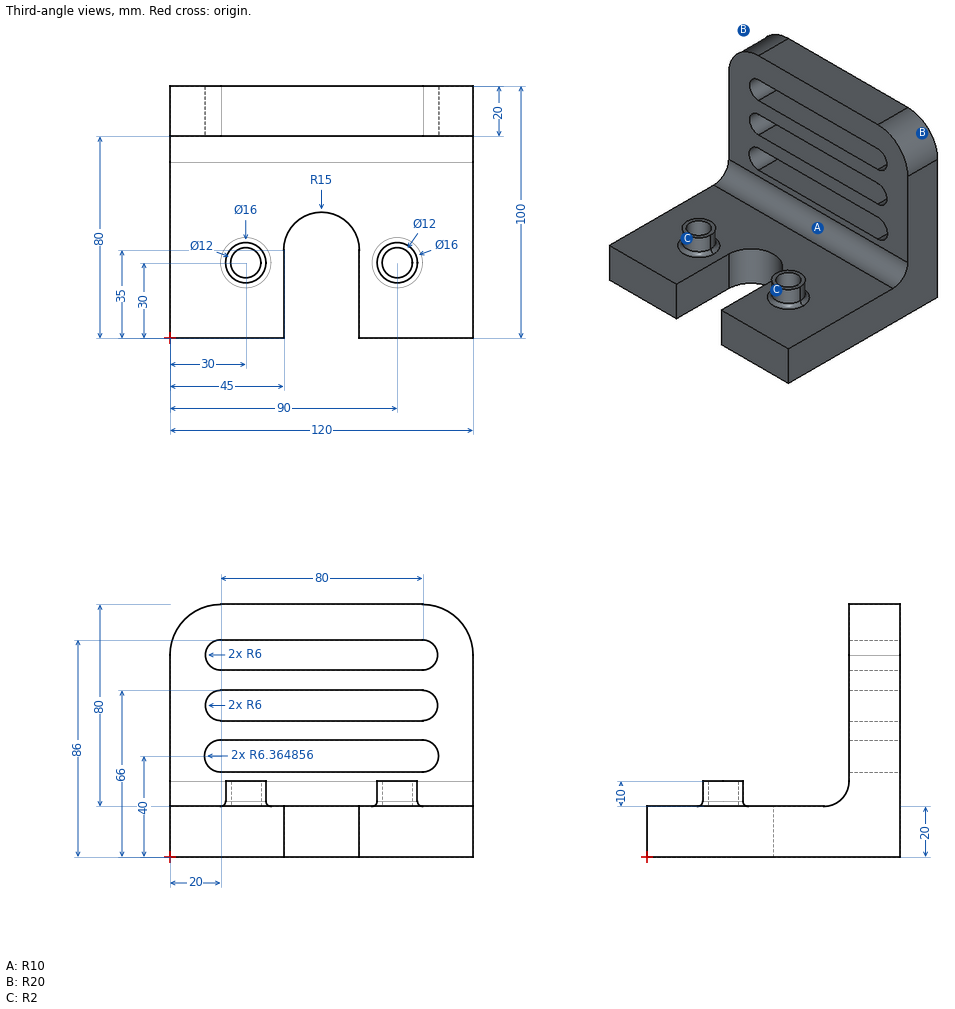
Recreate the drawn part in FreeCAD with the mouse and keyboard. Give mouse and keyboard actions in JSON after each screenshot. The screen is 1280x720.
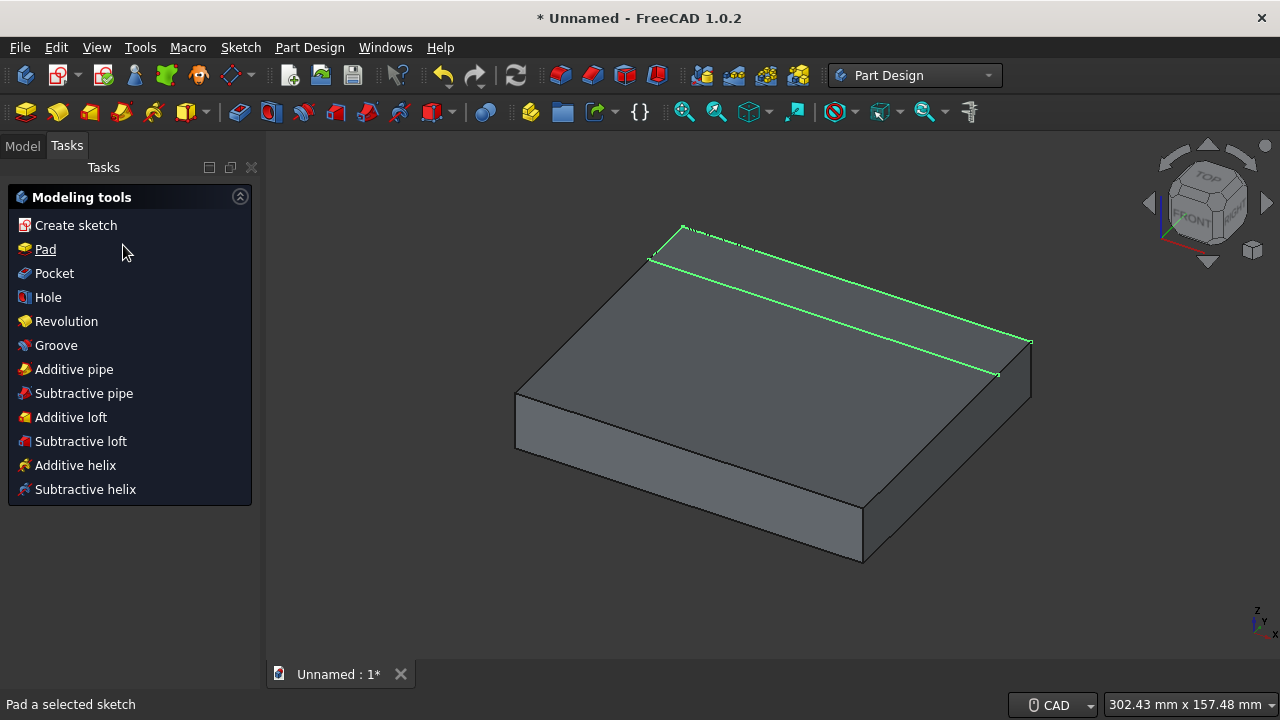
{"action": "left_click", "coordinate": [26, 112]}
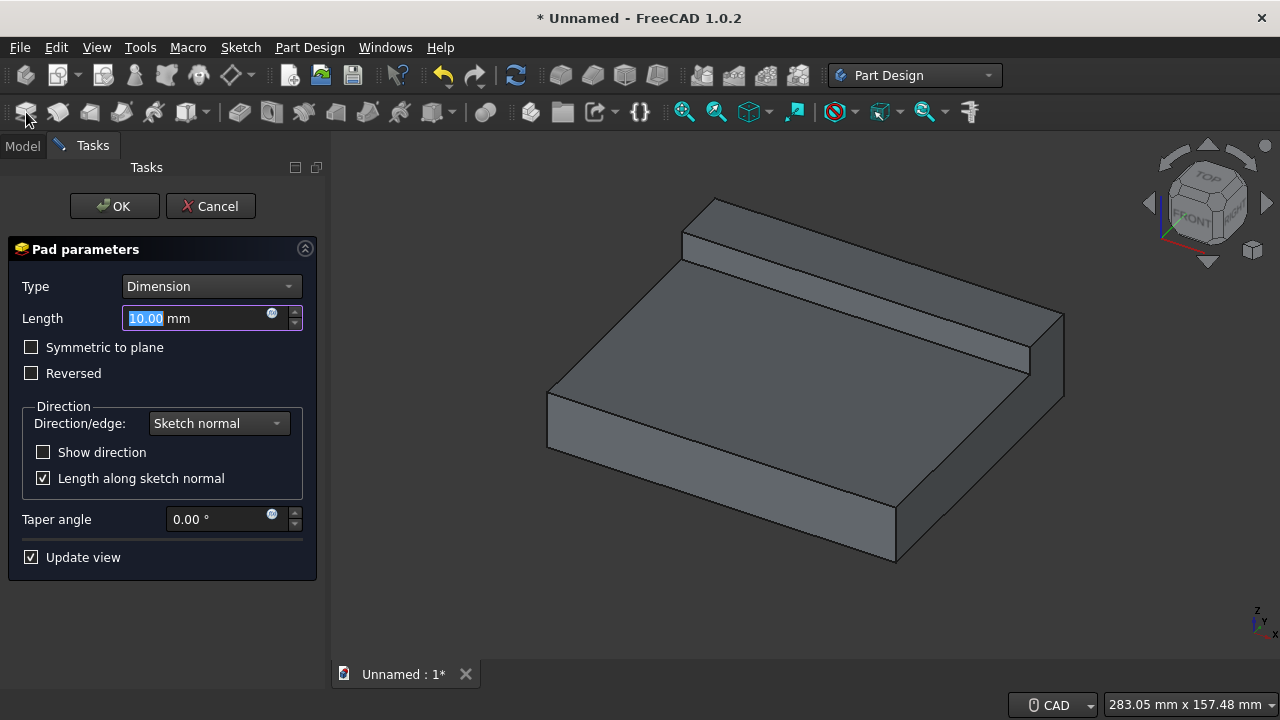
{"action": "type", "text": "80"}
{"action": "key", "text": "Tab"}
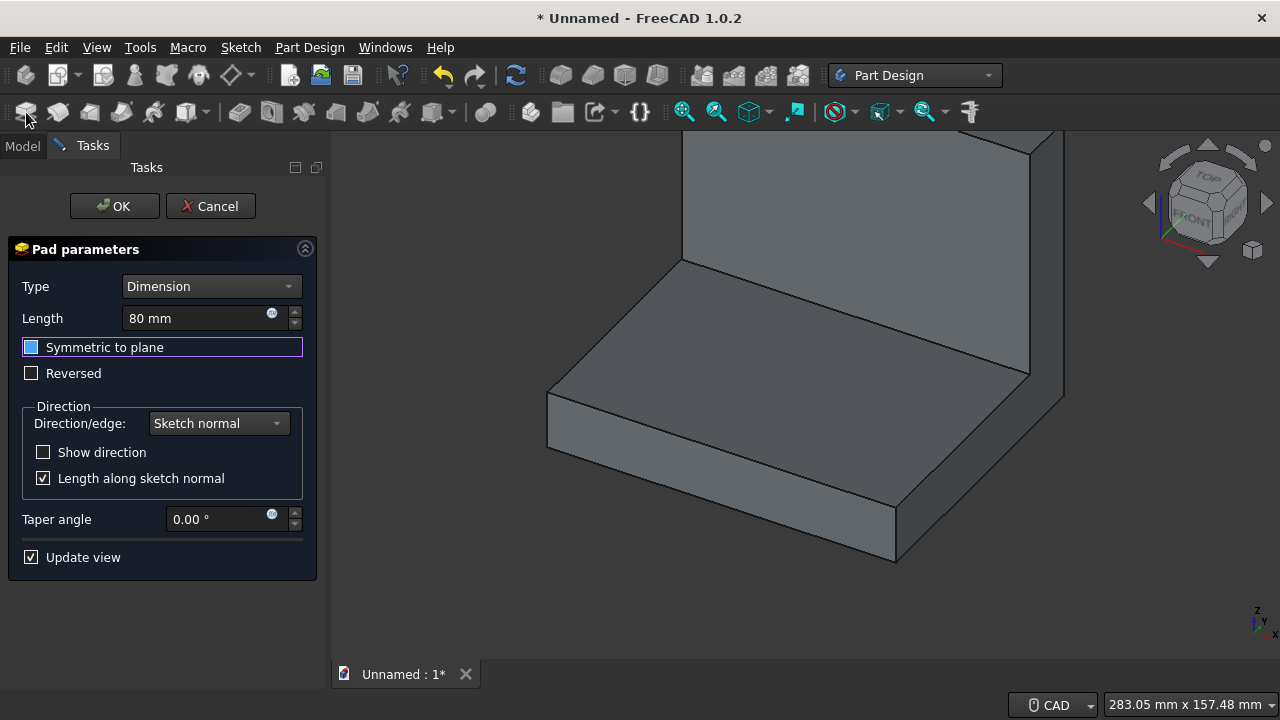
{"action": "left_click", "coordinate": [115, 206]}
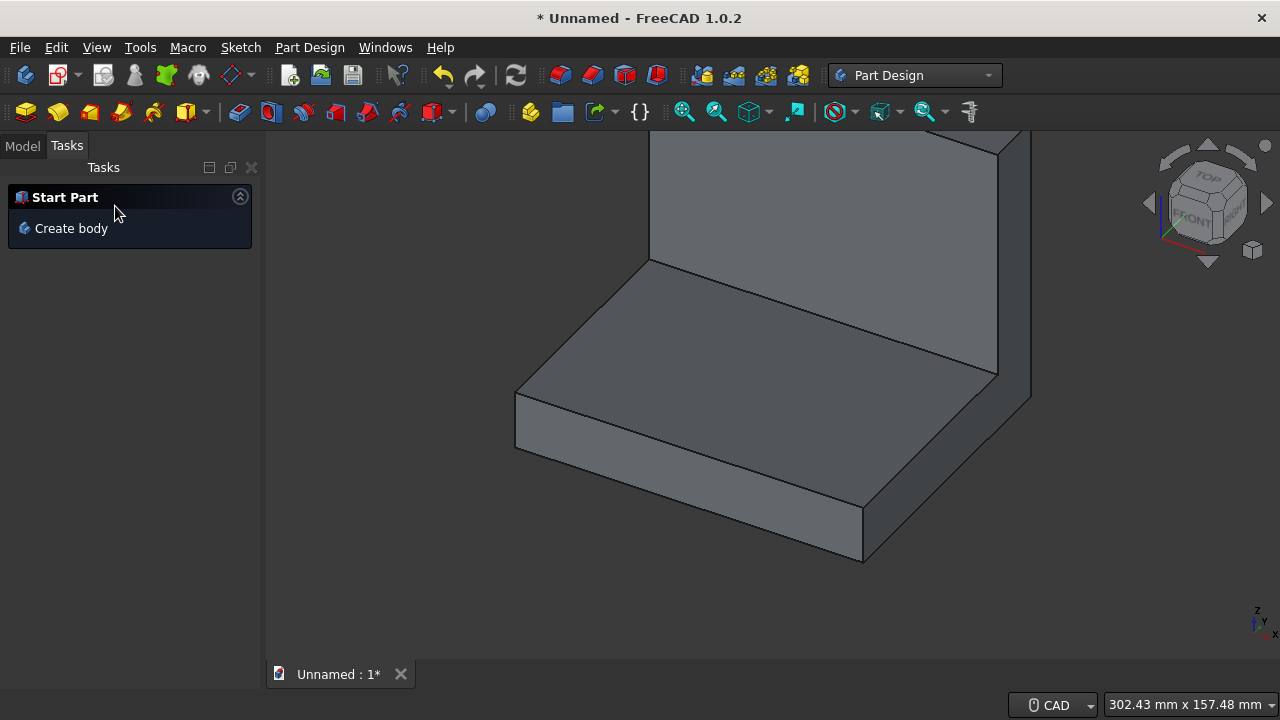
{"action": "key", "text": "v f"}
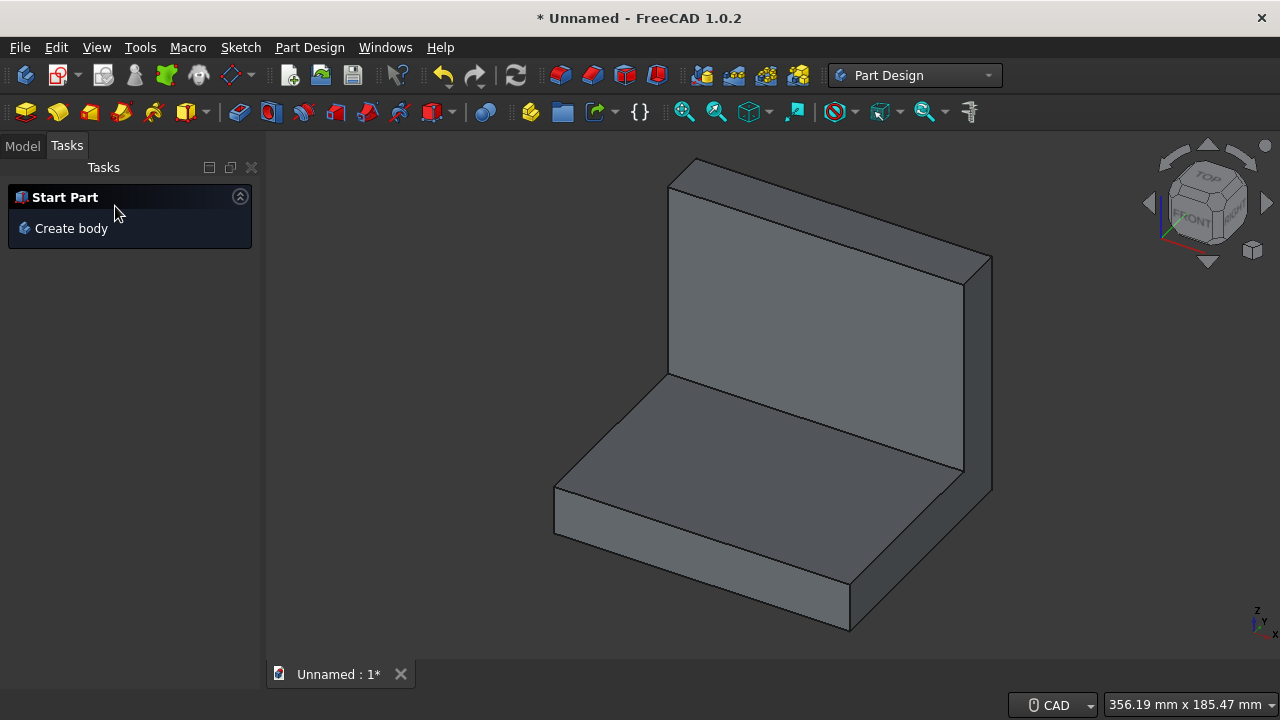
{"action": "left_click", "coordinate": [858, 342]}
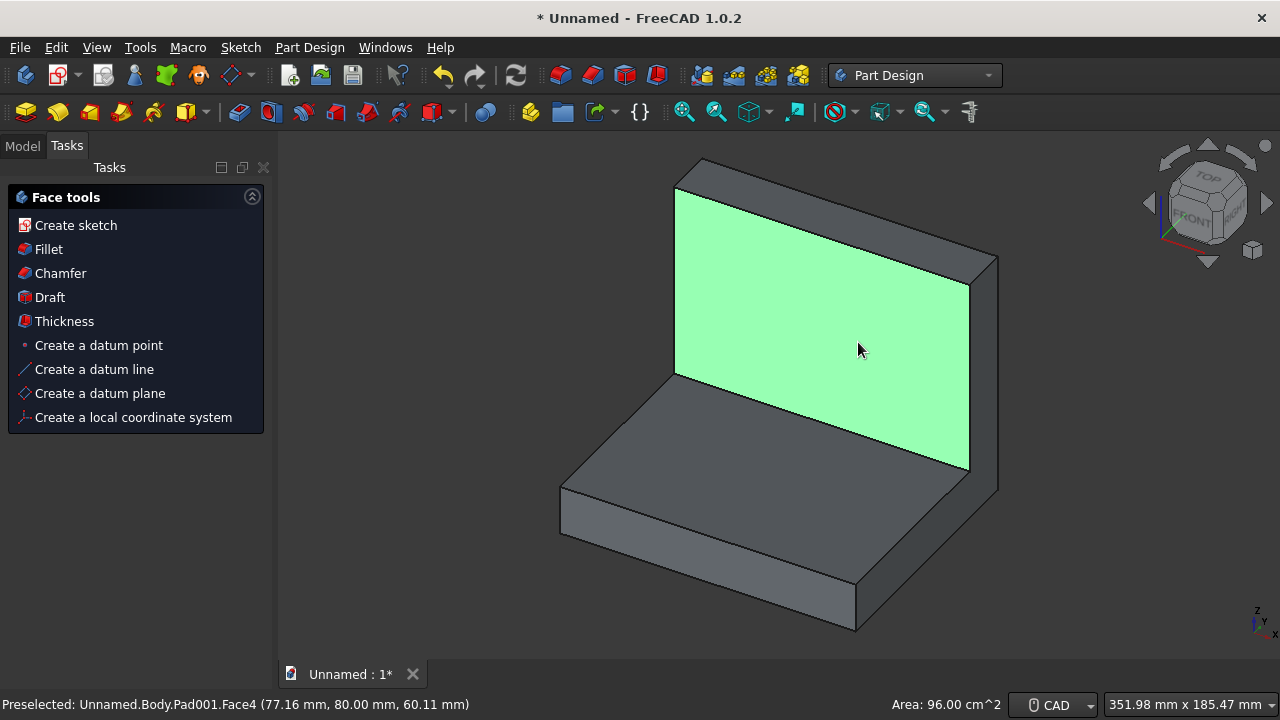
{"action": "left_click", "coordinate": [58, 76]}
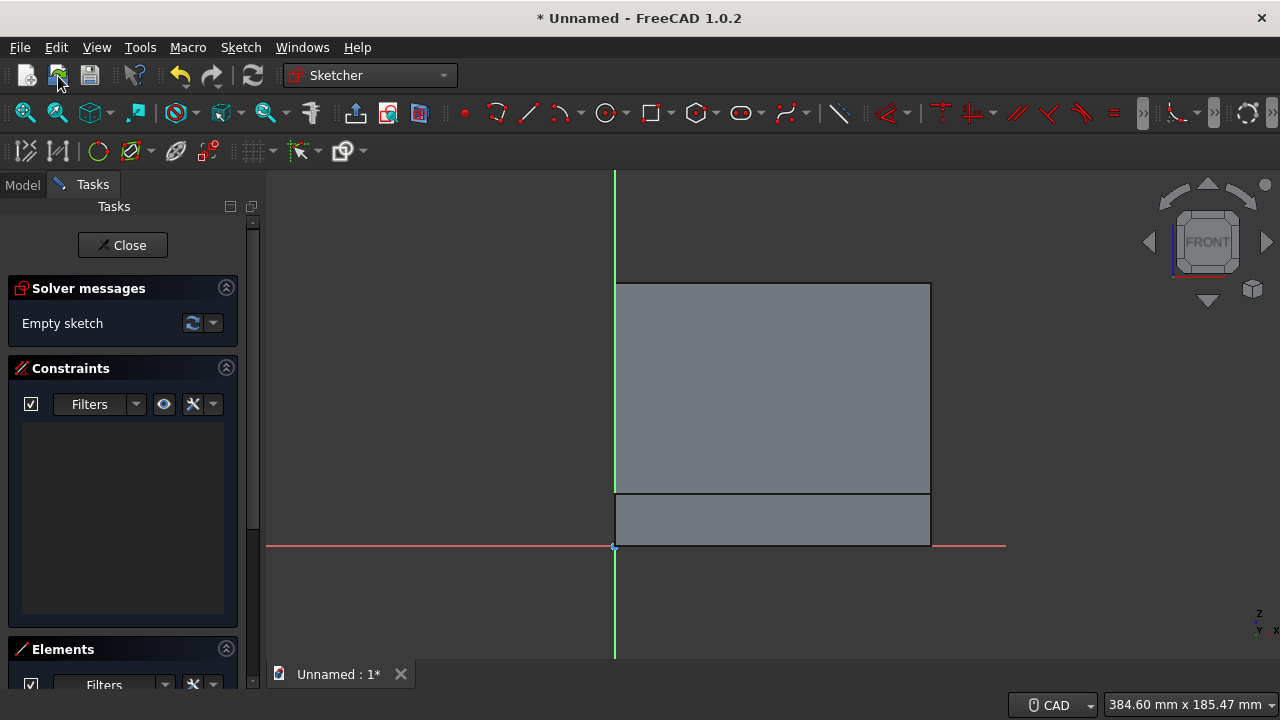
{"action": "key", "text": "g s"}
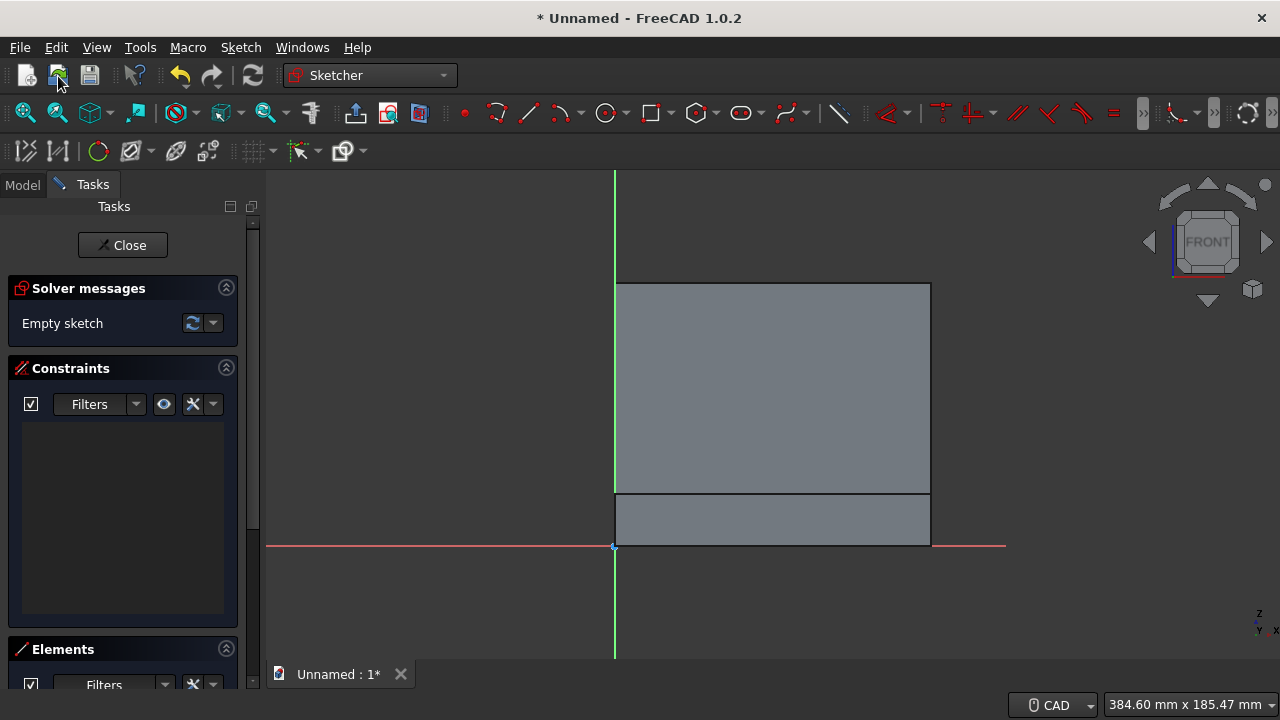
{"action": "scroll", "coordinate": [668, 335], "scroll_direction": "up", "scroll_amount": 2}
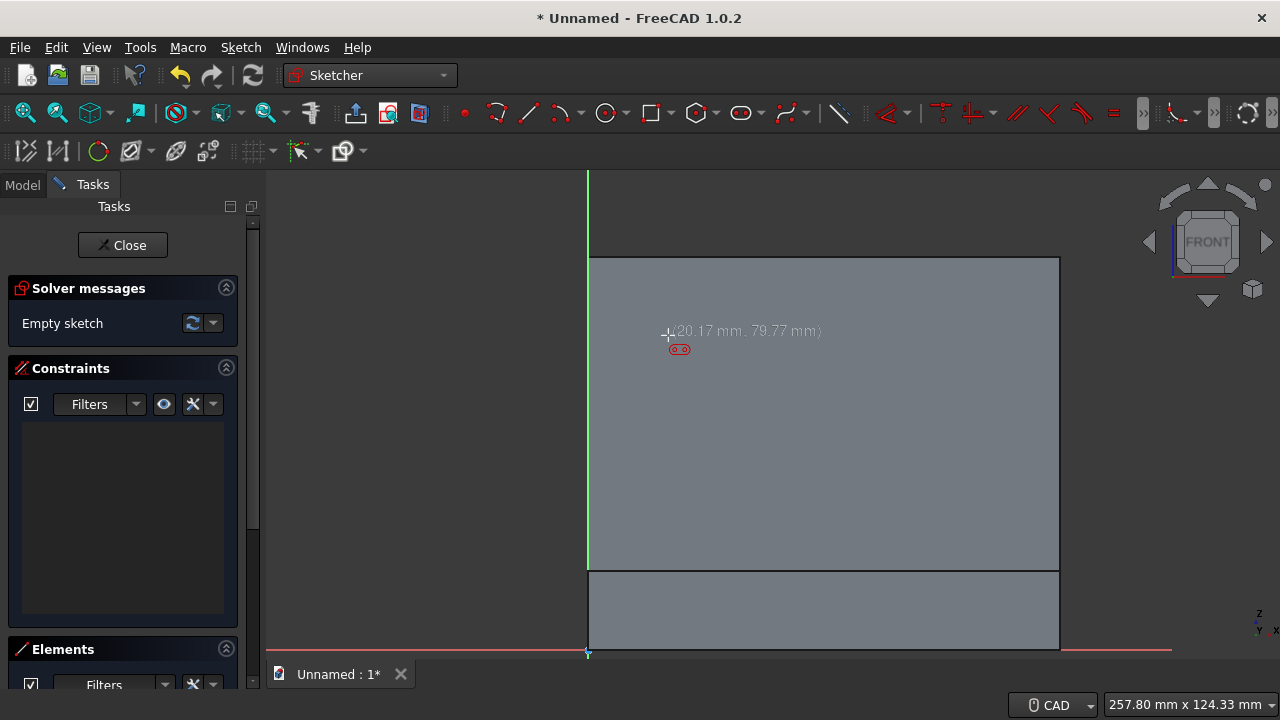
{"action": "left_click", "coordinate": [667, 335]}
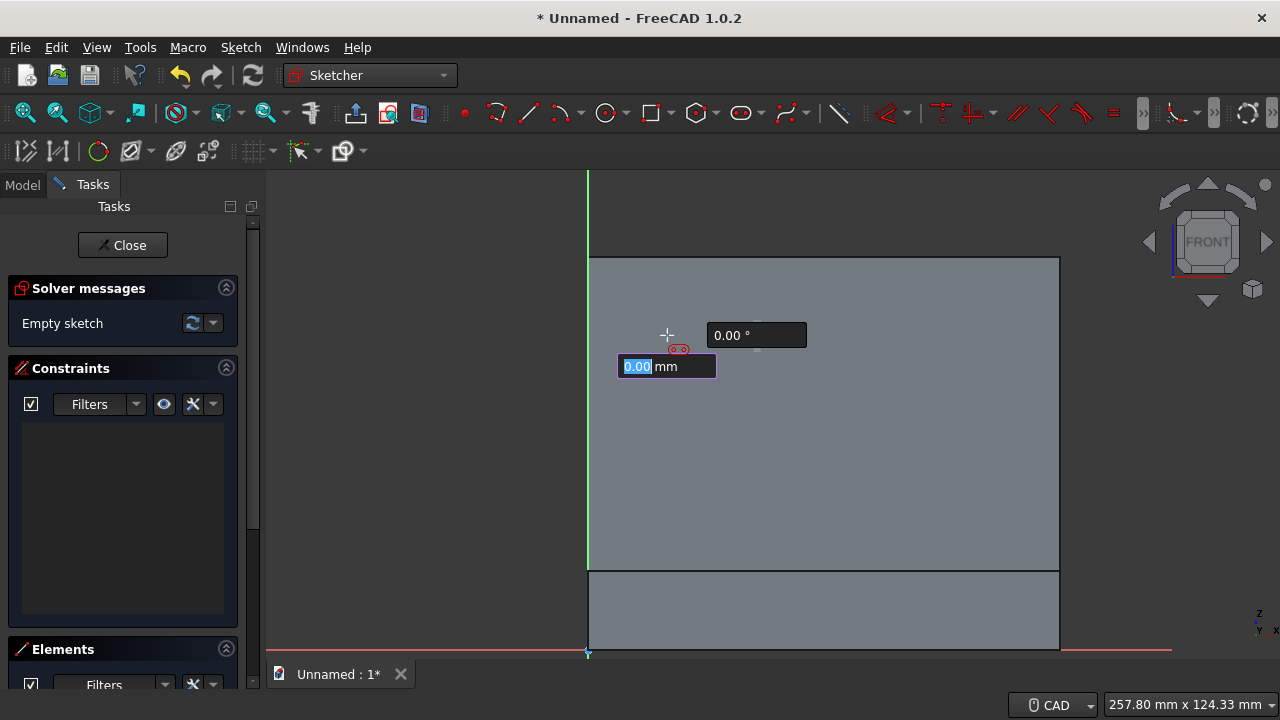
{"action": "left_click", "coordinate": [982, 335]}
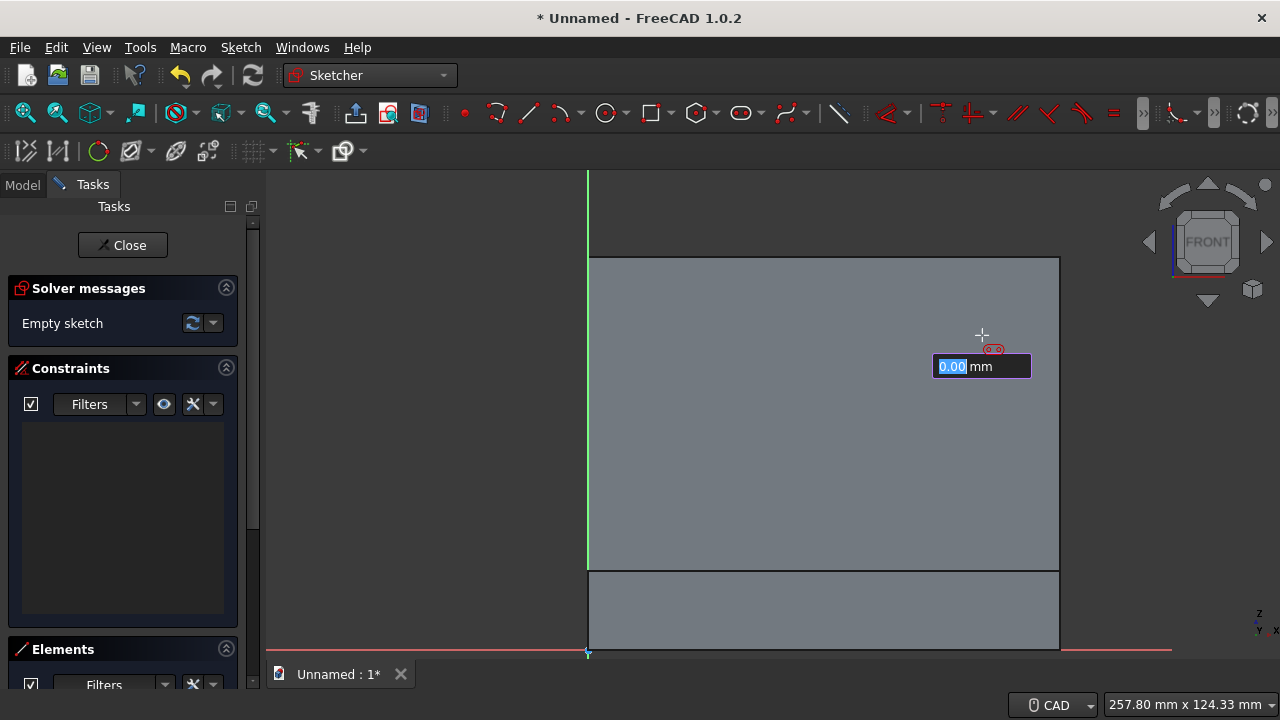
{"action": "left_click", "coordinate": [824, 312]}
{"action": "key", "text": "Escape"}